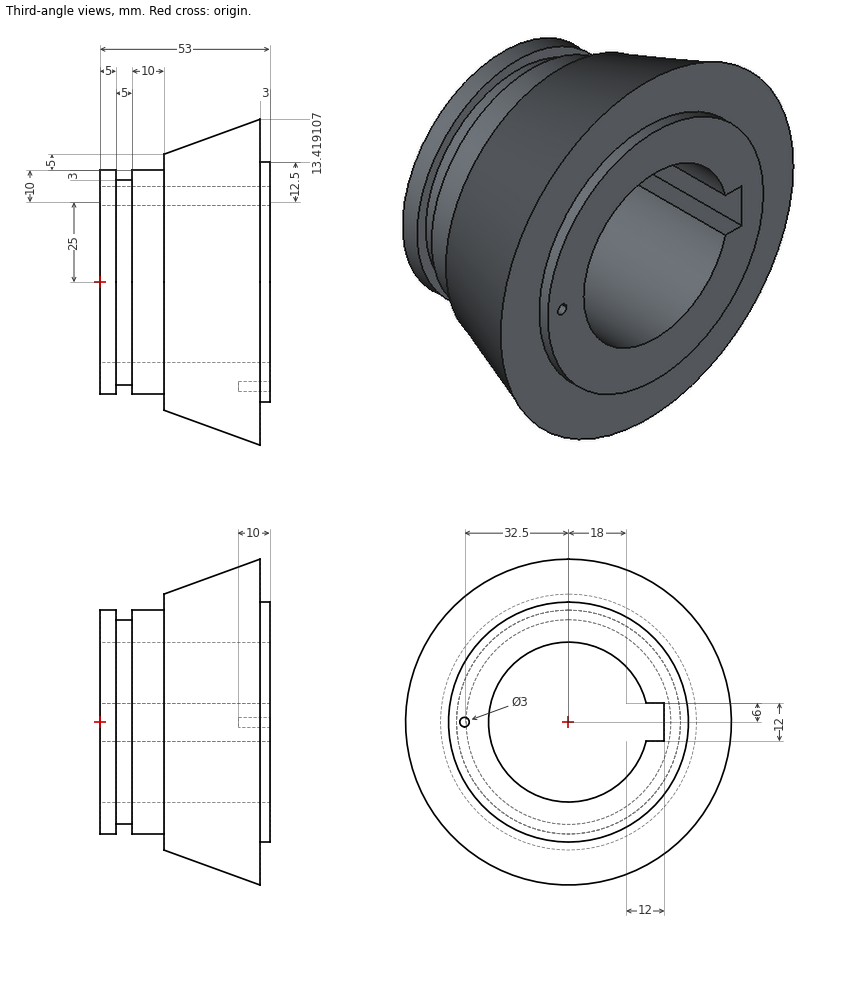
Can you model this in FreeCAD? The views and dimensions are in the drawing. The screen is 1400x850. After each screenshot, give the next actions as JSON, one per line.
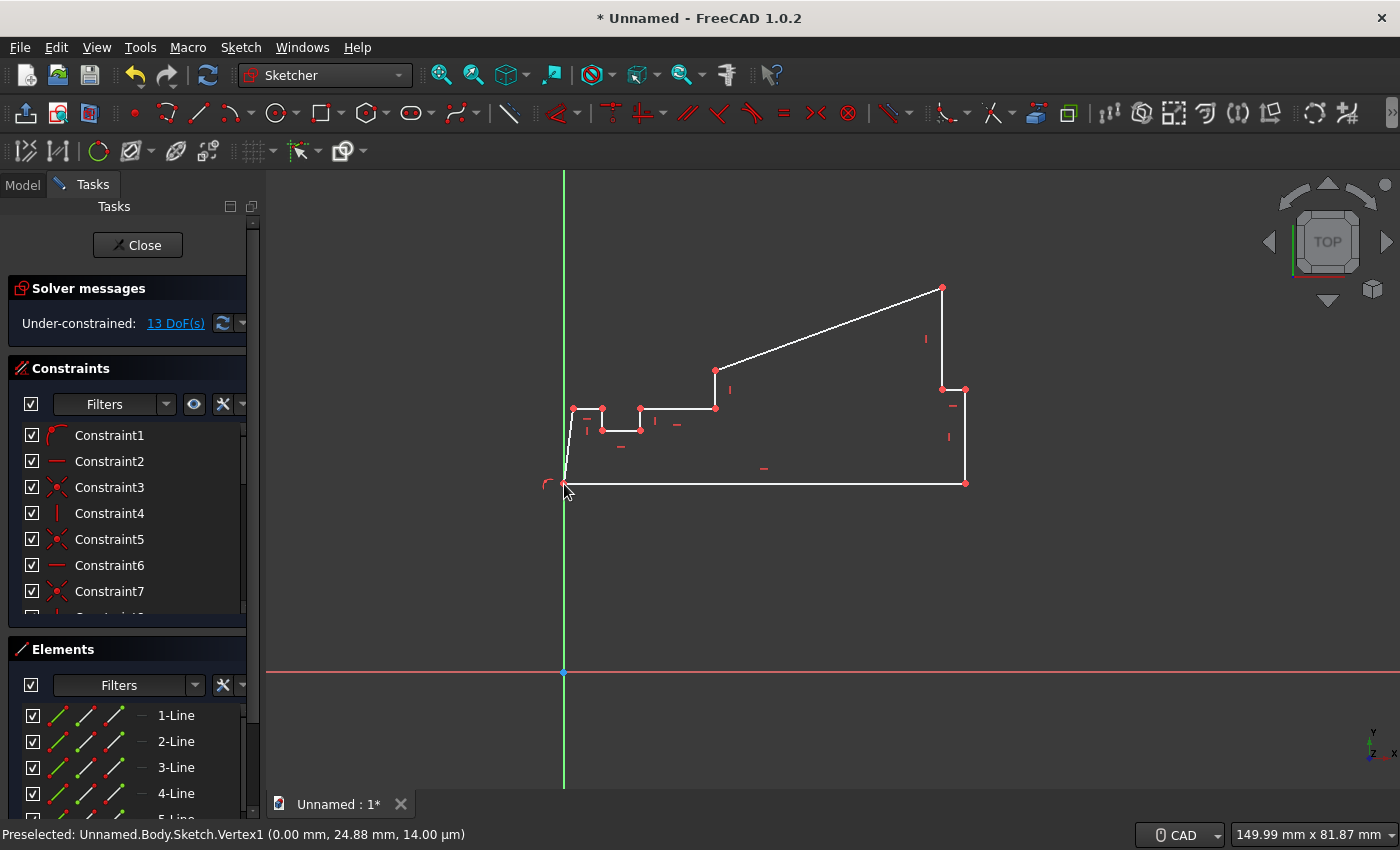
{"action": "left_click", "coordinate": [567, 462]}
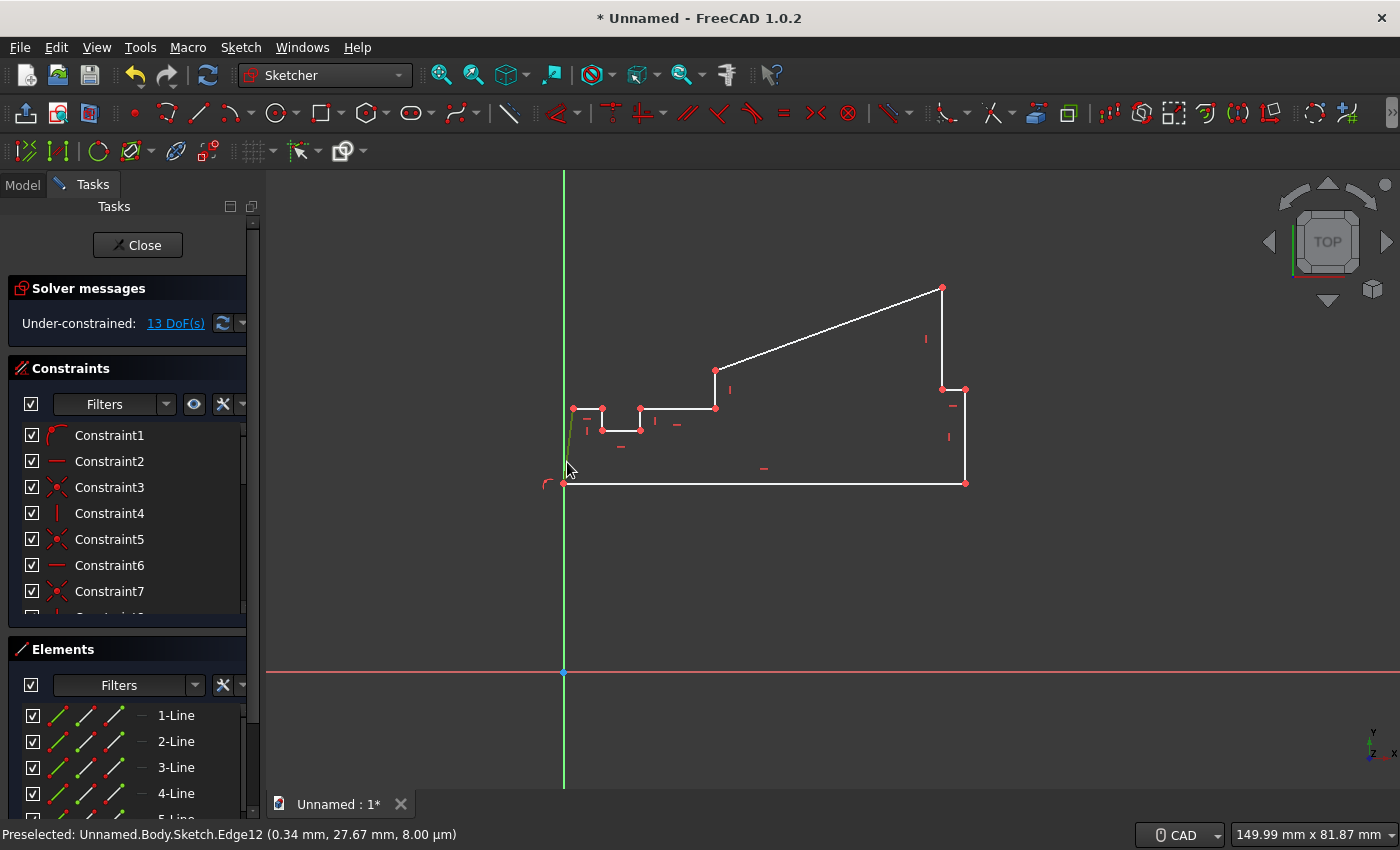
{"action": "left_click", "coordinate": [666, 114]}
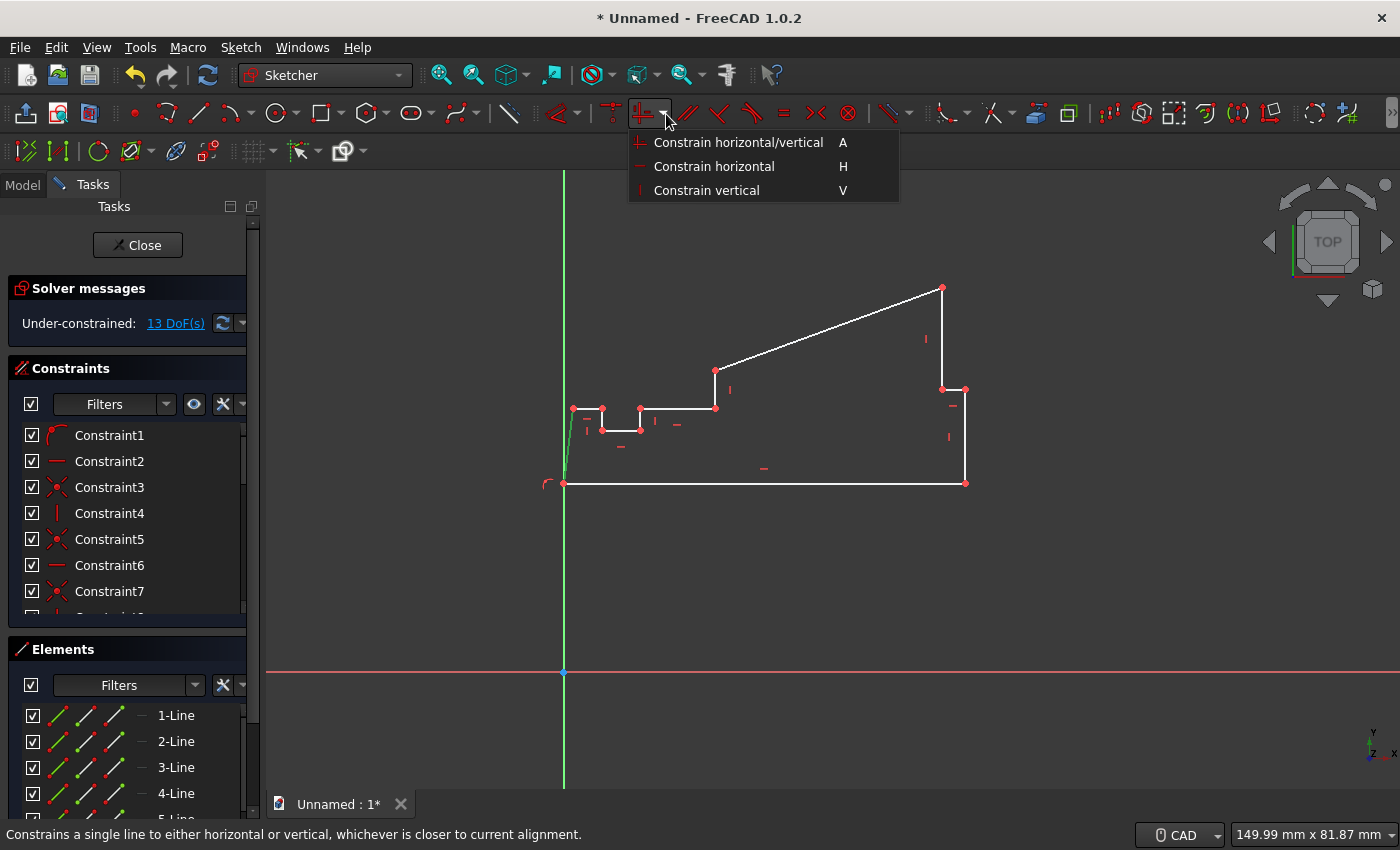
{"action": "left_click", "coordinate": [764, 190]}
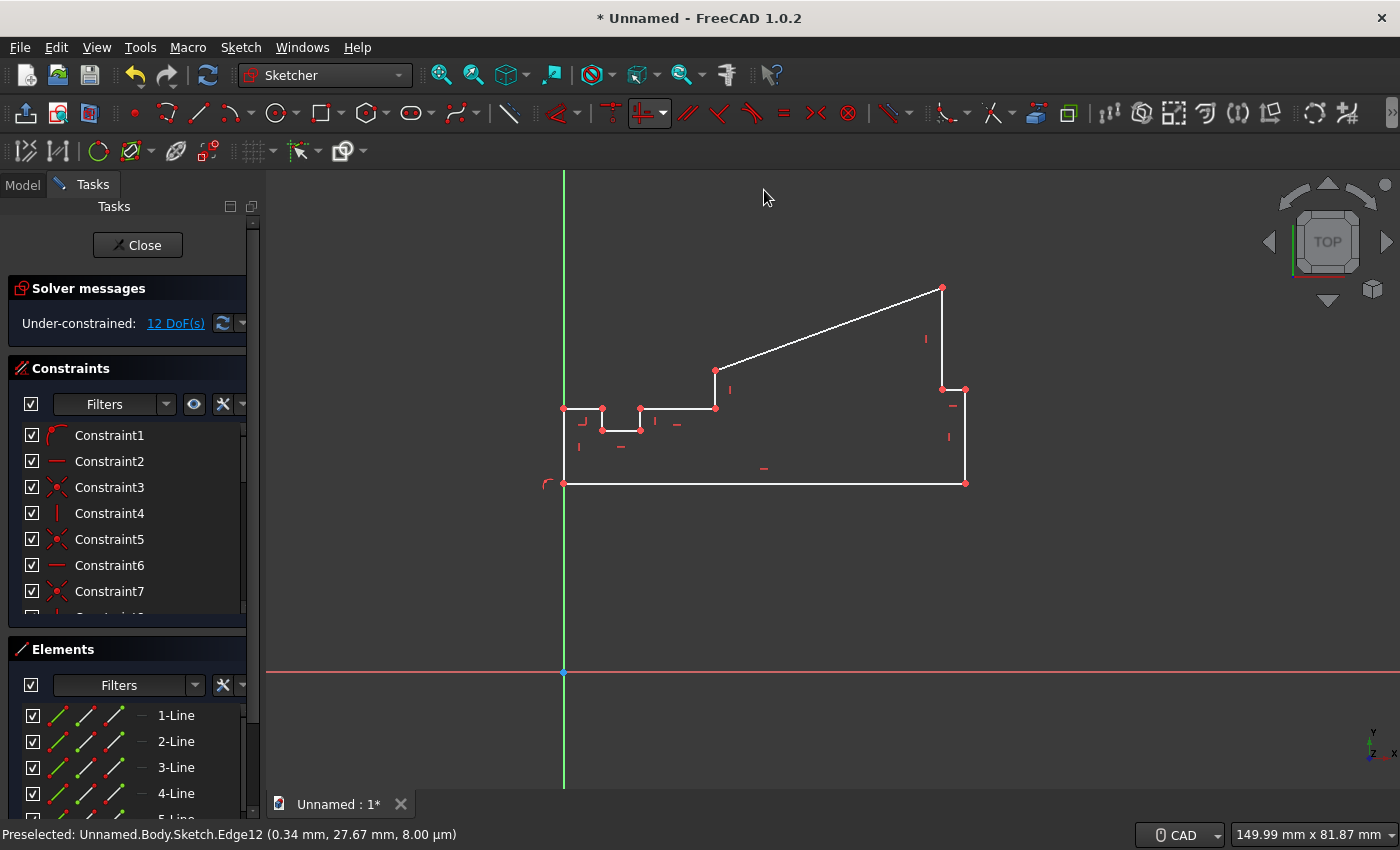
{"action": "left_click", "coordinate": [556, 114]}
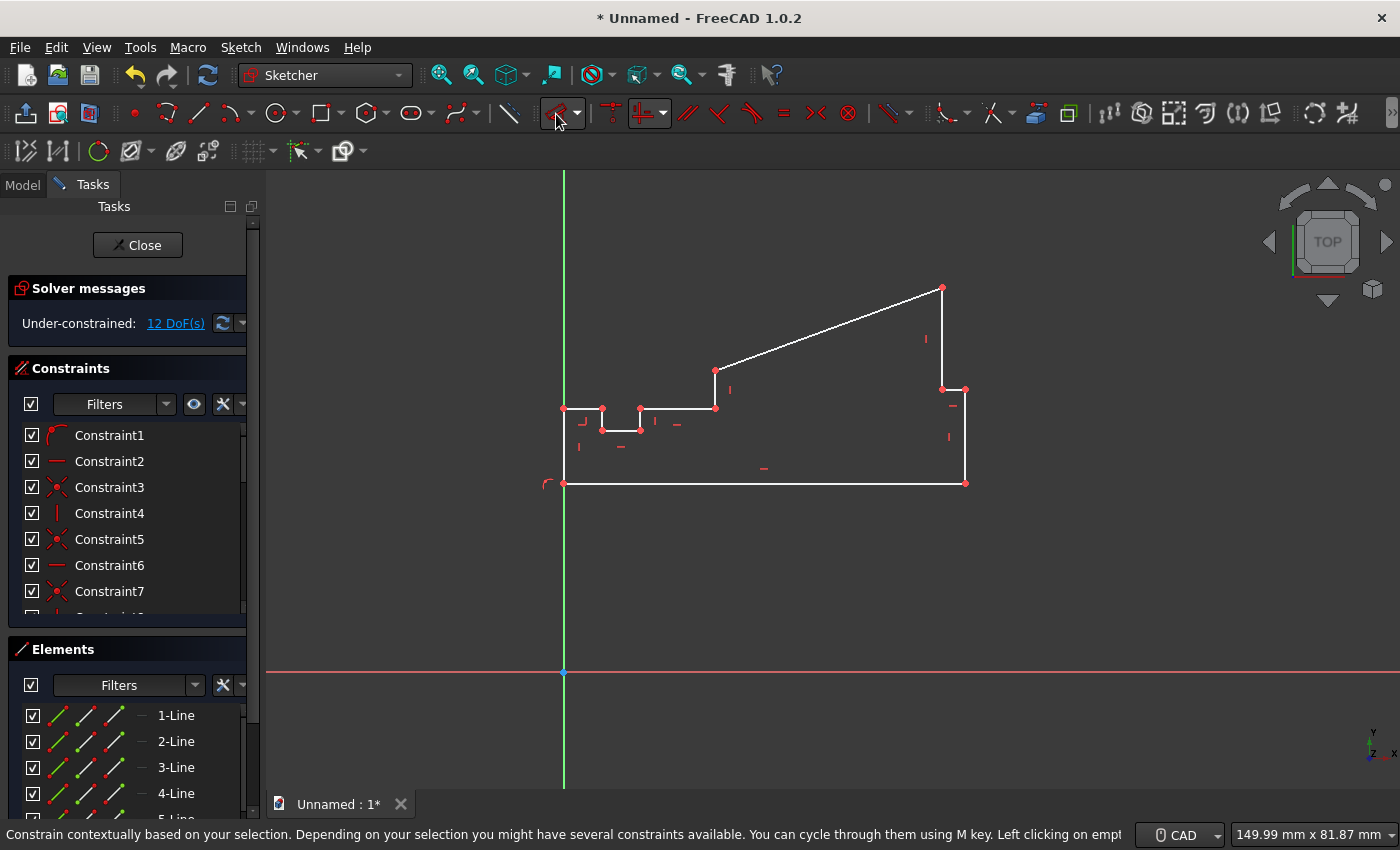
{"action": "scroll", "coordinate": [956, 390], "scroll_direction": "up", "scroll_amount": 3}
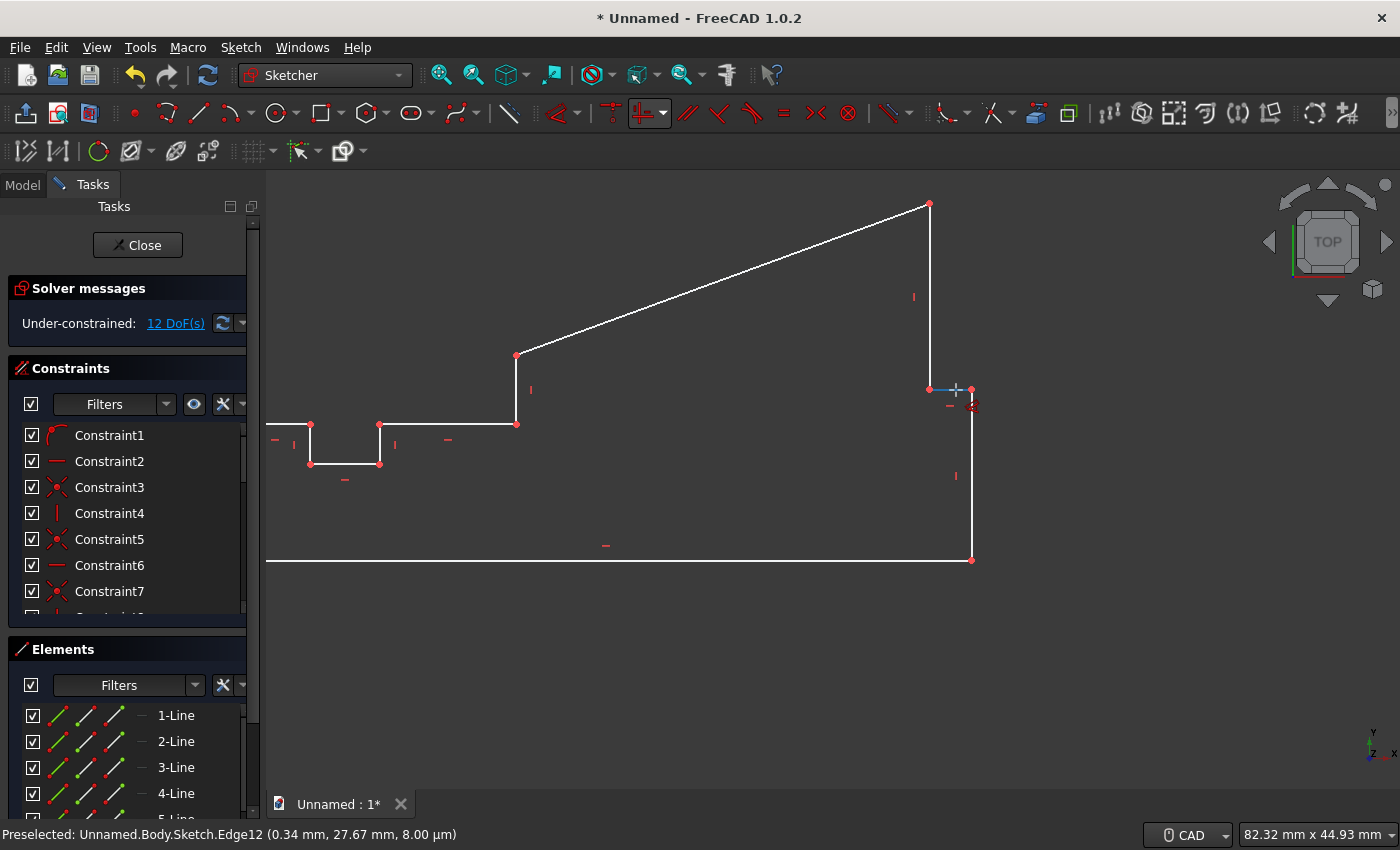
{"action": "left_click", "coordinate": [955, 390]}
{"action": "left_click", "coordinate": [951, 356]}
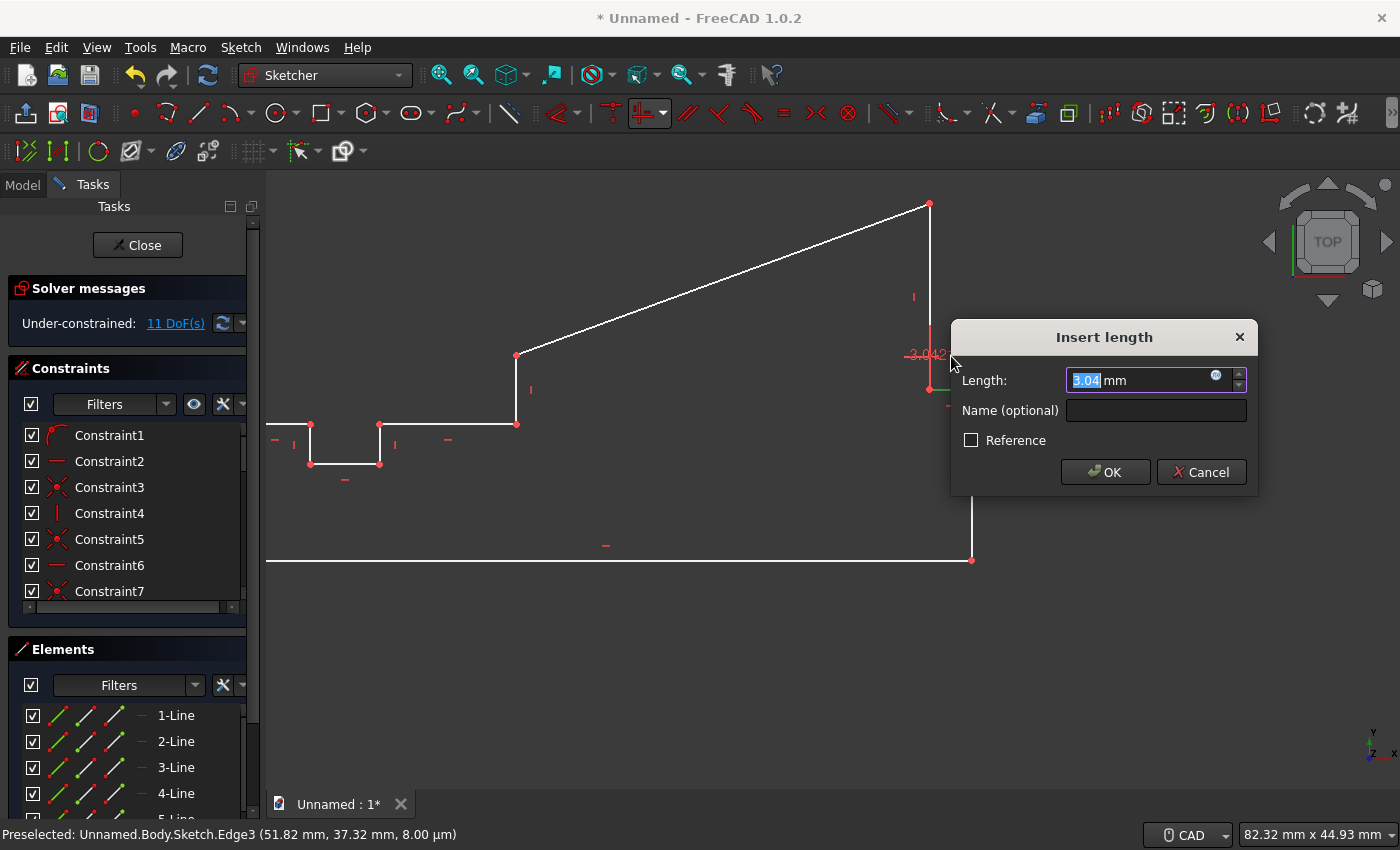
{"action": "type", "text": "3"}
{"action": "key", "text": "Return"}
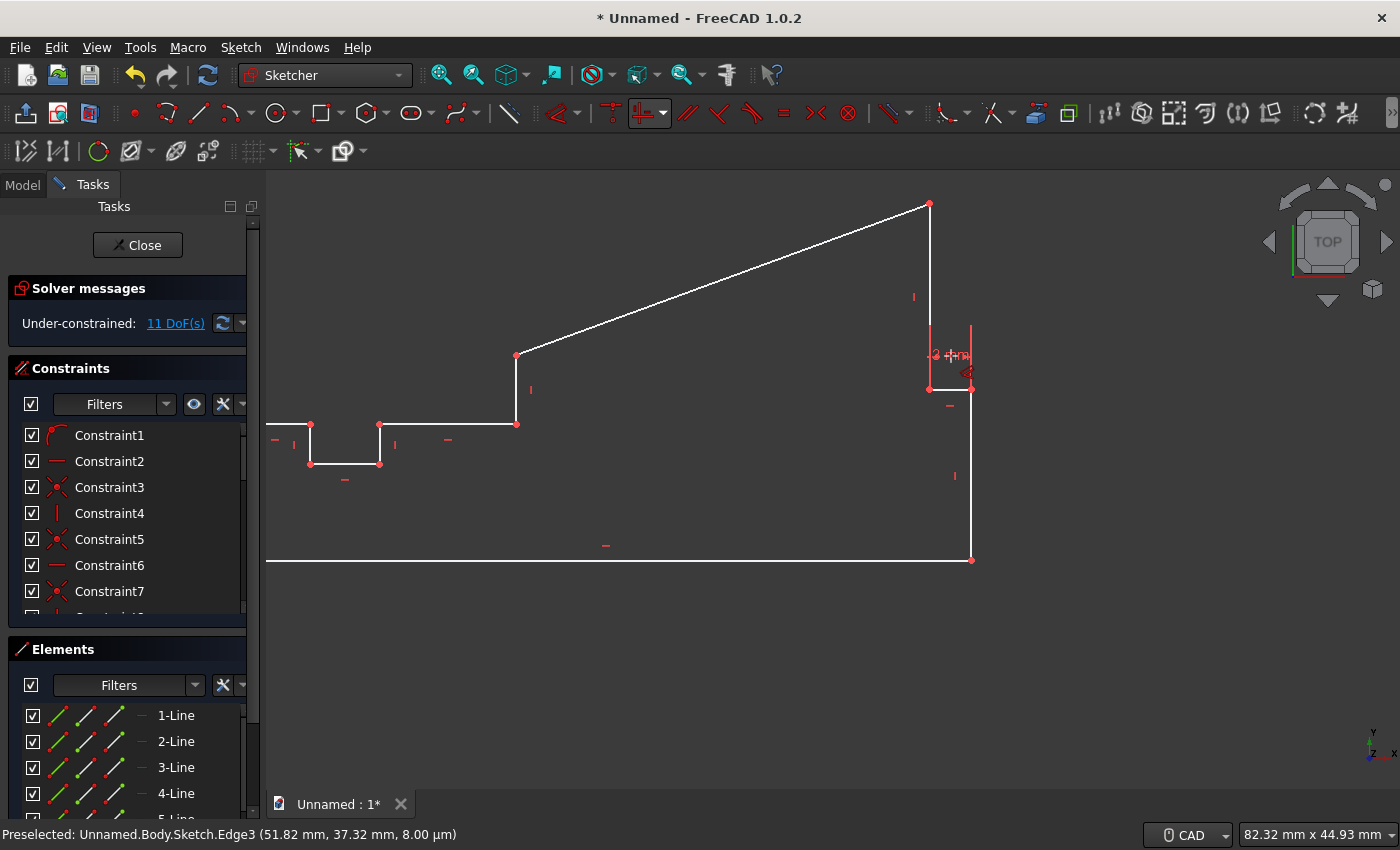
{"action": "left_click", "coordinate": [516, 376]}
{"action": "left_click", "coordinate": [482, 390]}